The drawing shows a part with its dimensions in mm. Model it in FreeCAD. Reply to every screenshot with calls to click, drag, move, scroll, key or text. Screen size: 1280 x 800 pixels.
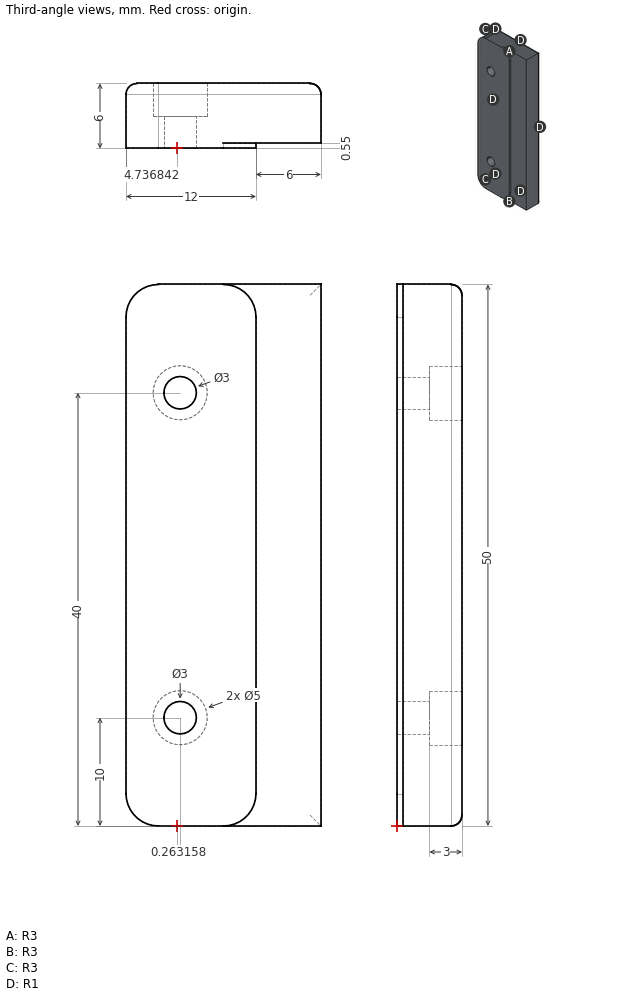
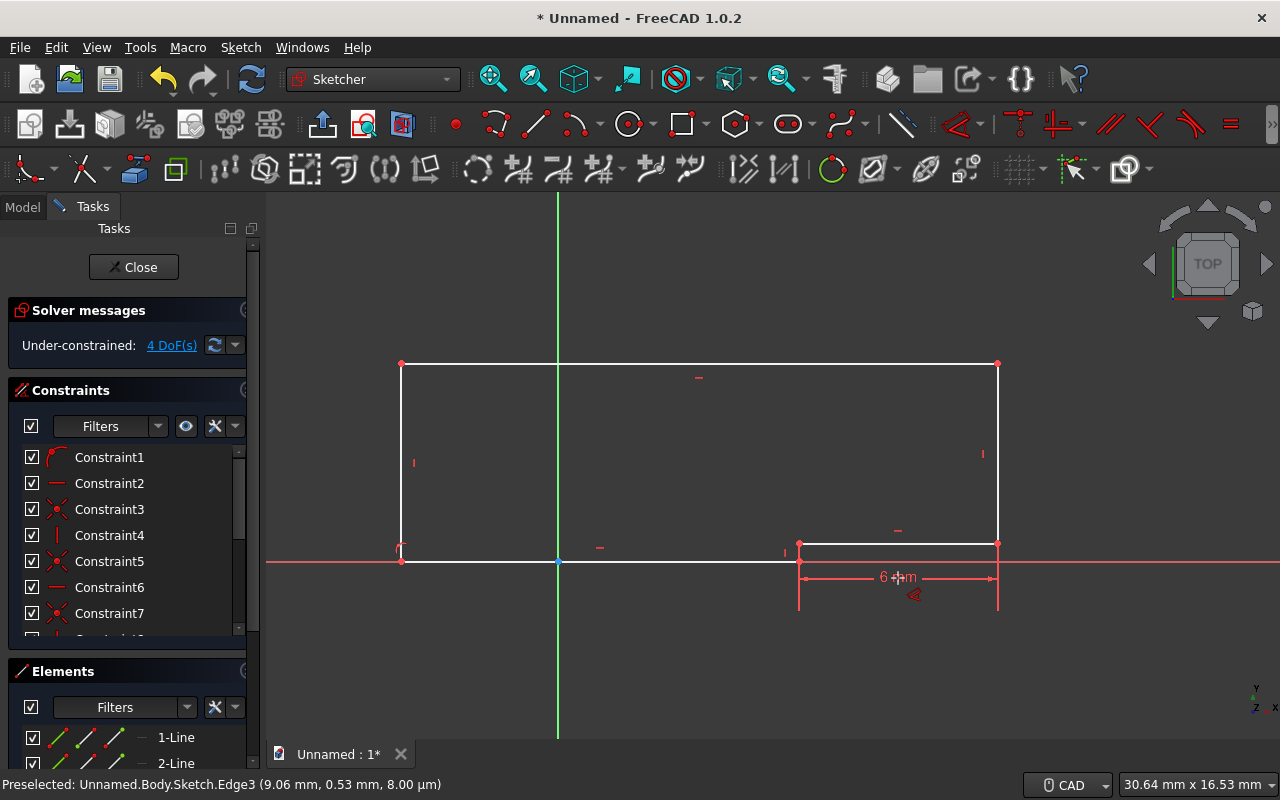
click(401, 423)
click(367, 463)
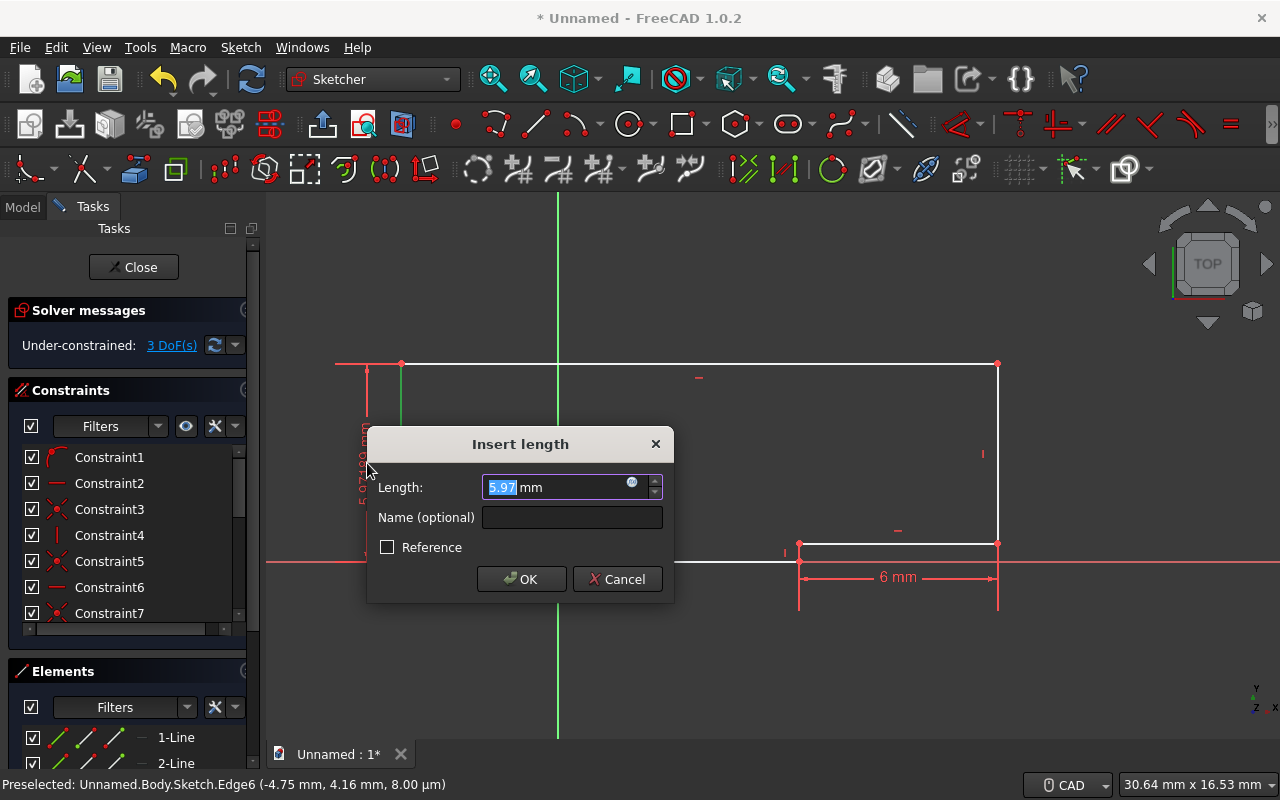
text(6)
key(Return)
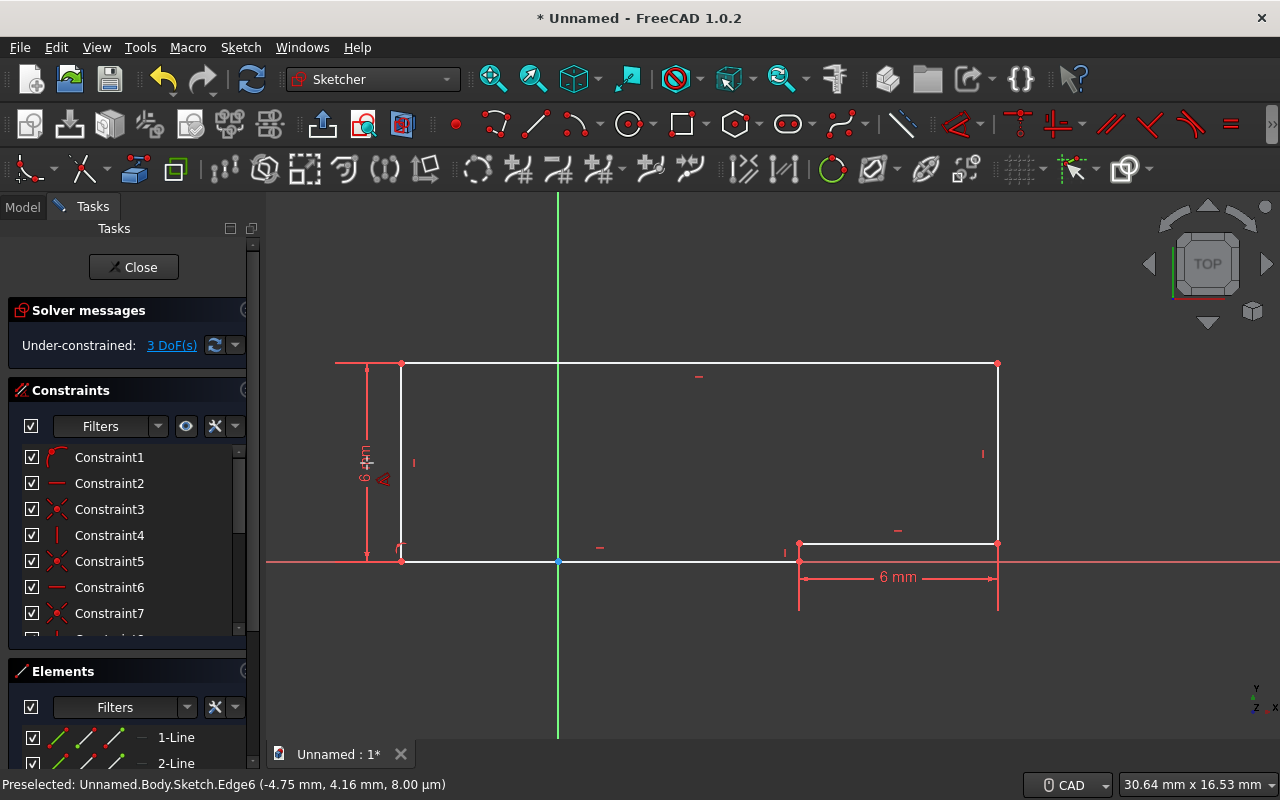
click(520, 562)
click(600, 596)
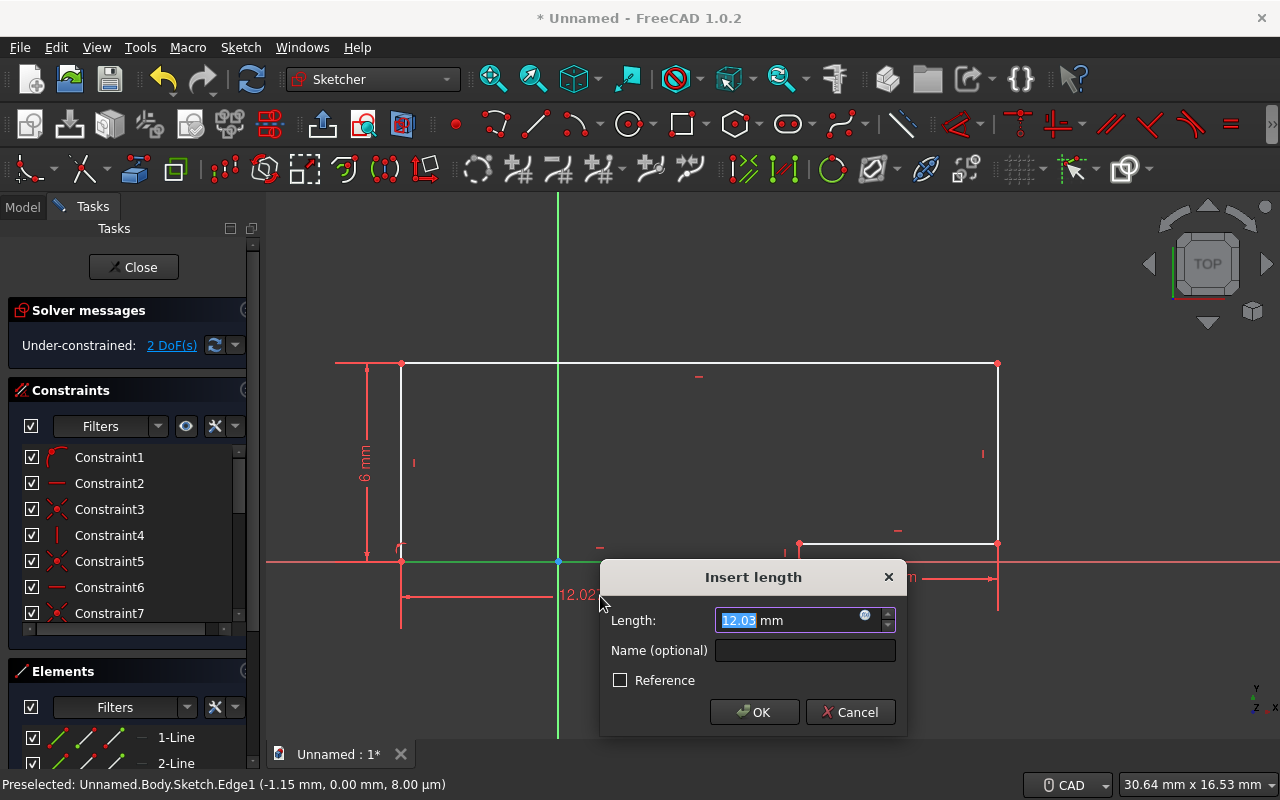
text(12)
key(Return)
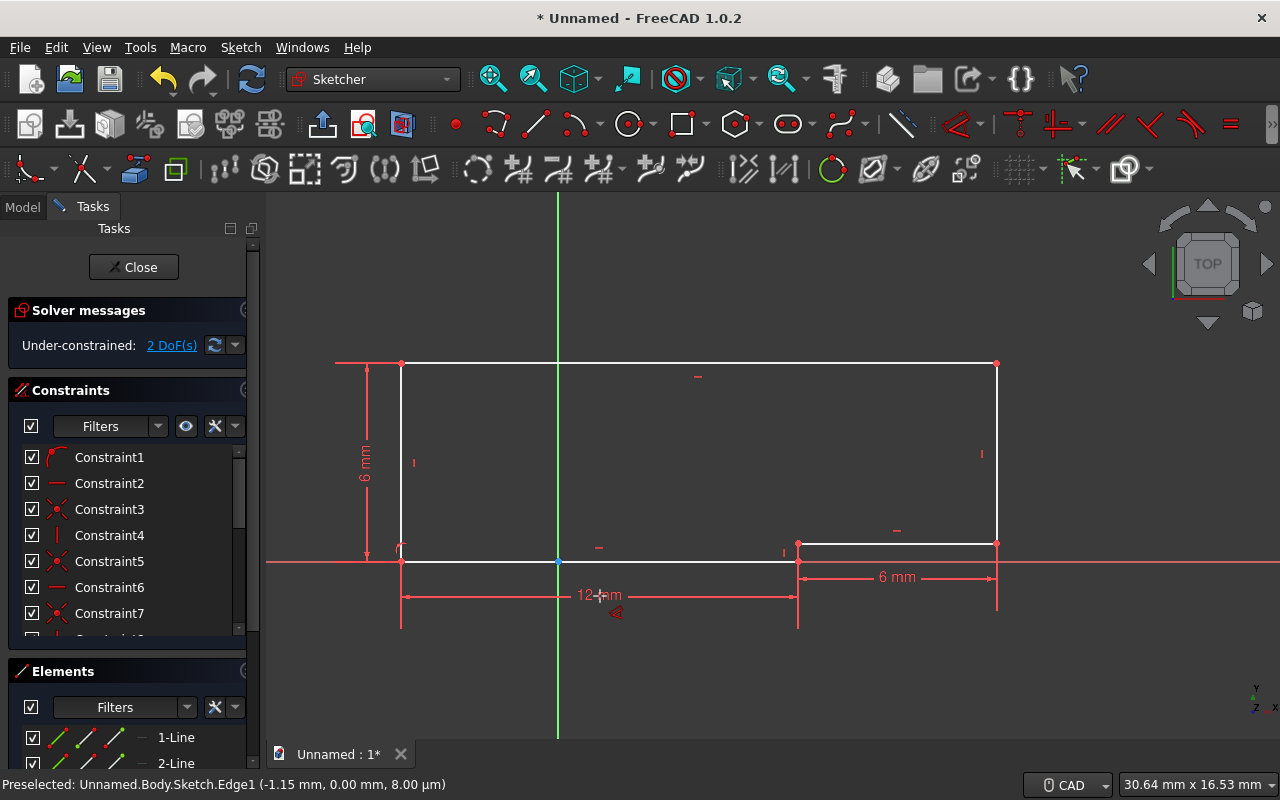
scroll(798, 553, up, 4)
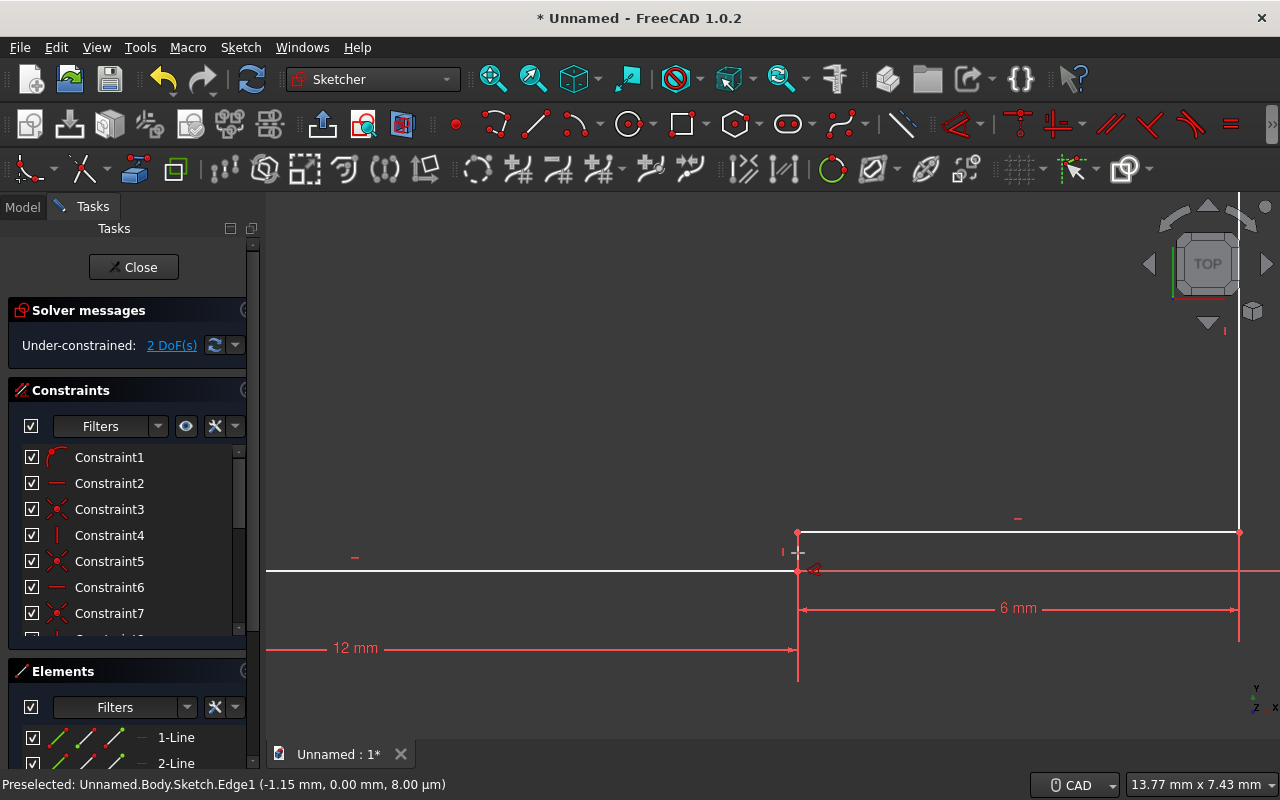
click(798, 552)
click(832, 552)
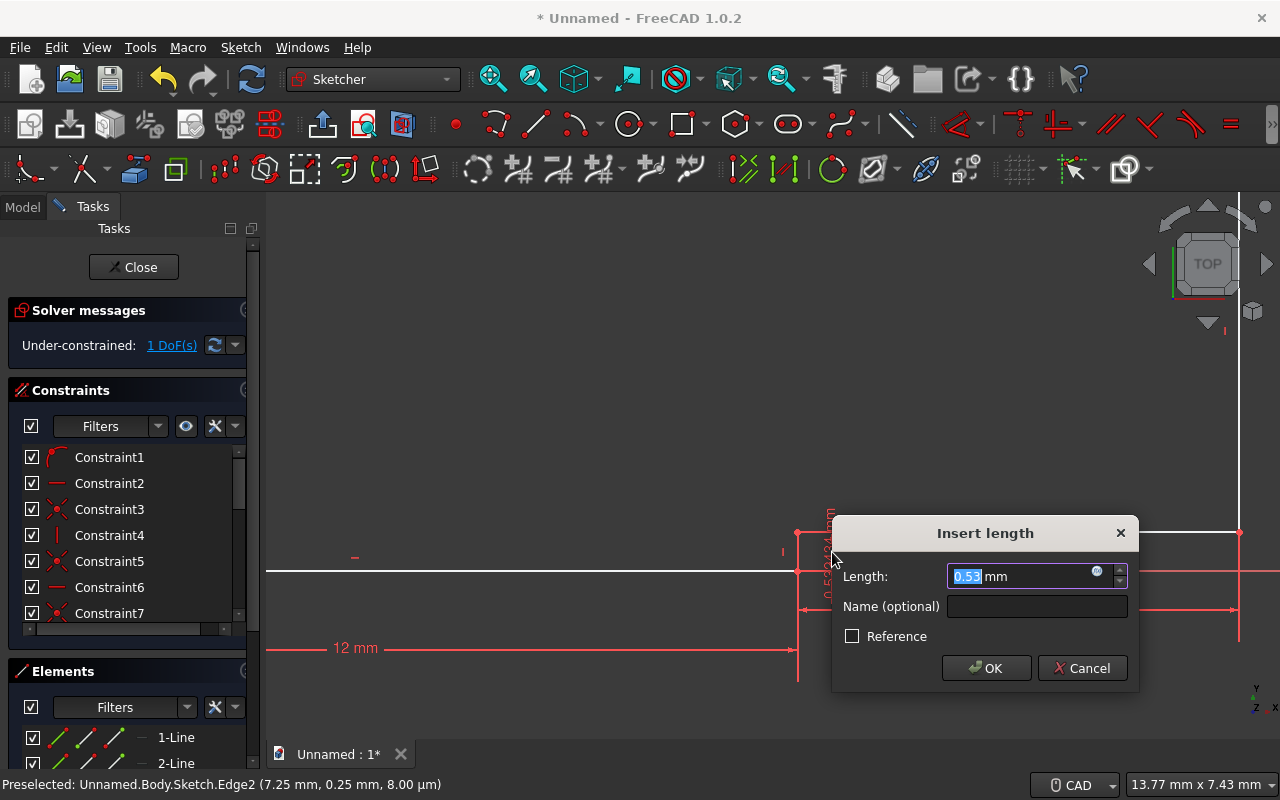
text(0.55)
key(Return)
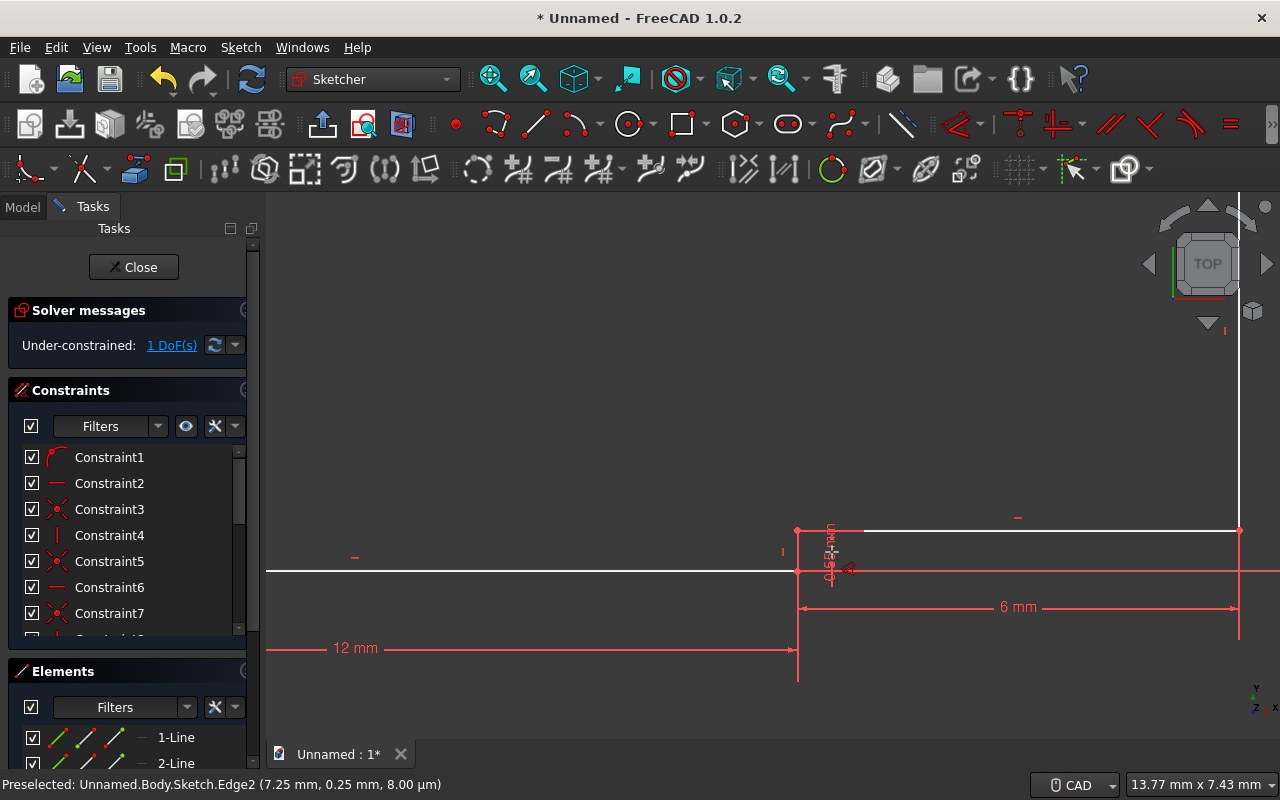
scroll(808, 559, down, 4)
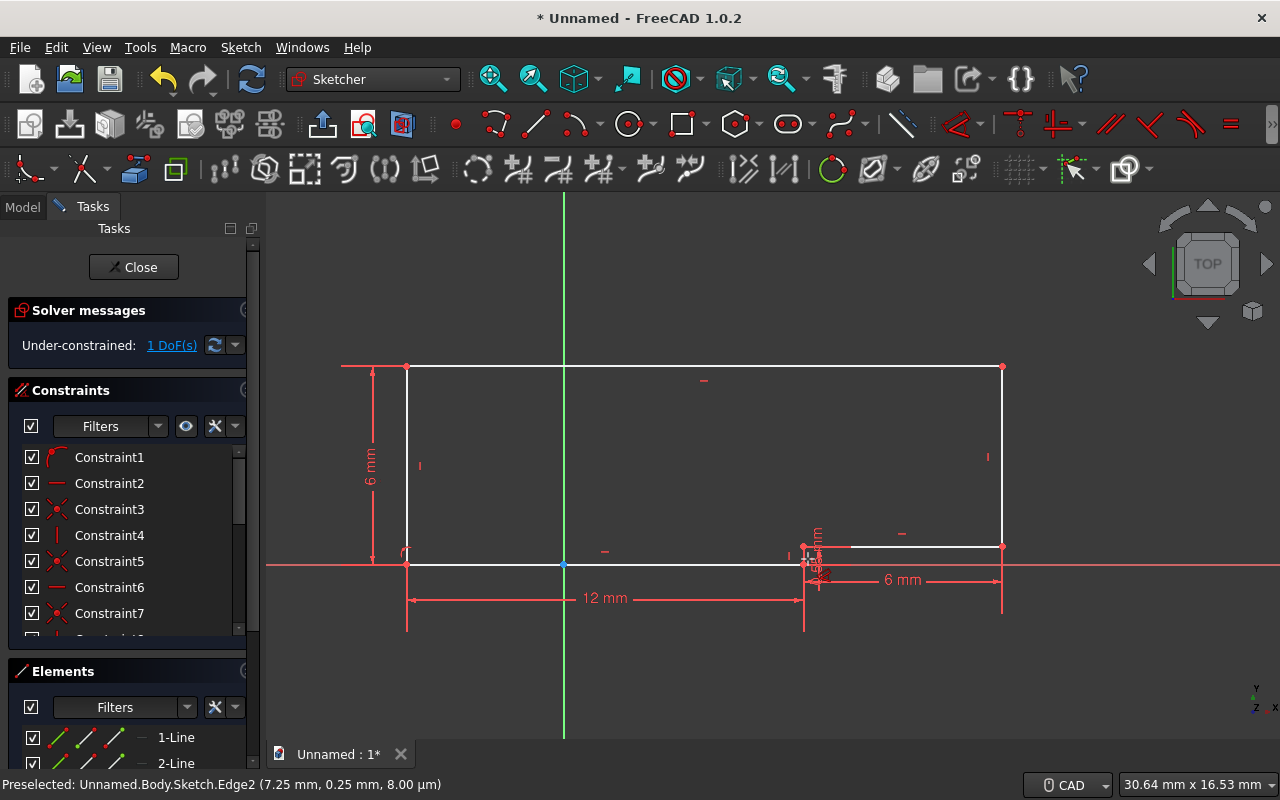
click(407, 565)
click(485, 599)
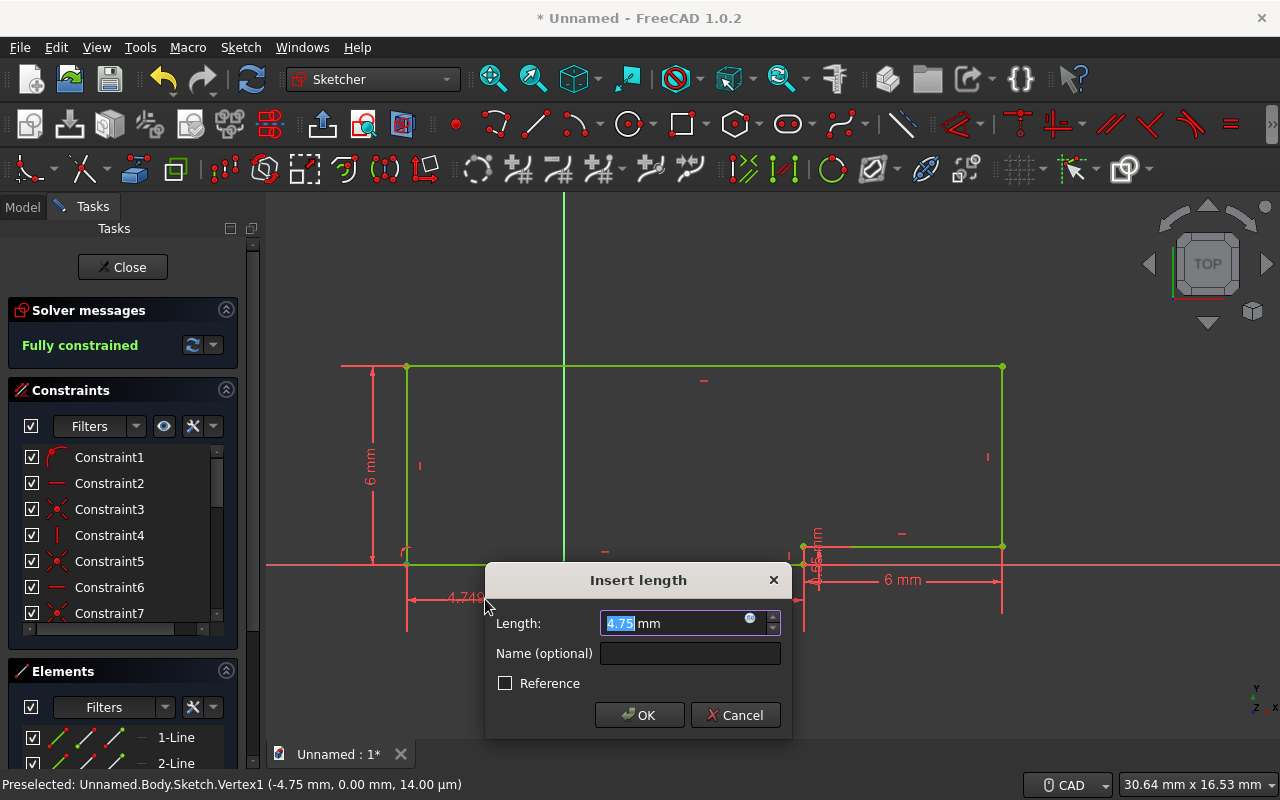
text(4.736842)
key(Return)
key(Escape)